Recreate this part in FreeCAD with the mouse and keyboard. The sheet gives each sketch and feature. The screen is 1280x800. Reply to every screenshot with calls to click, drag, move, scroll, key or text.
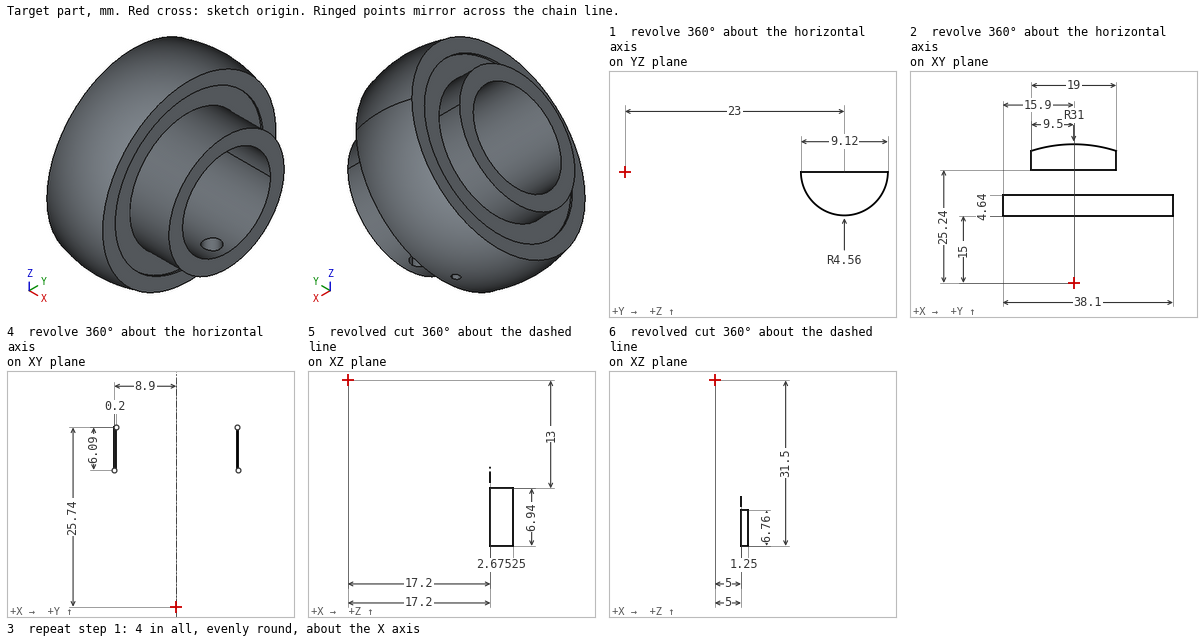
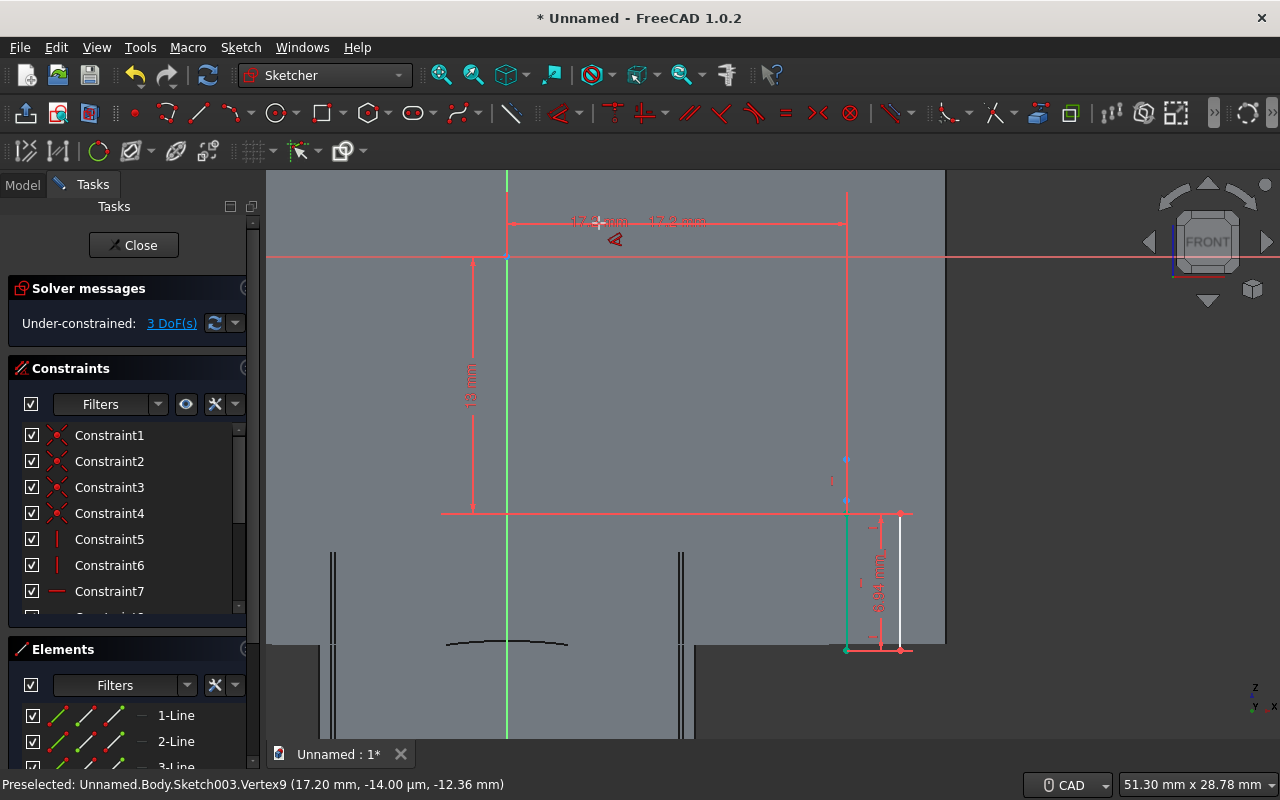
click(863, 651)
click(873, 685)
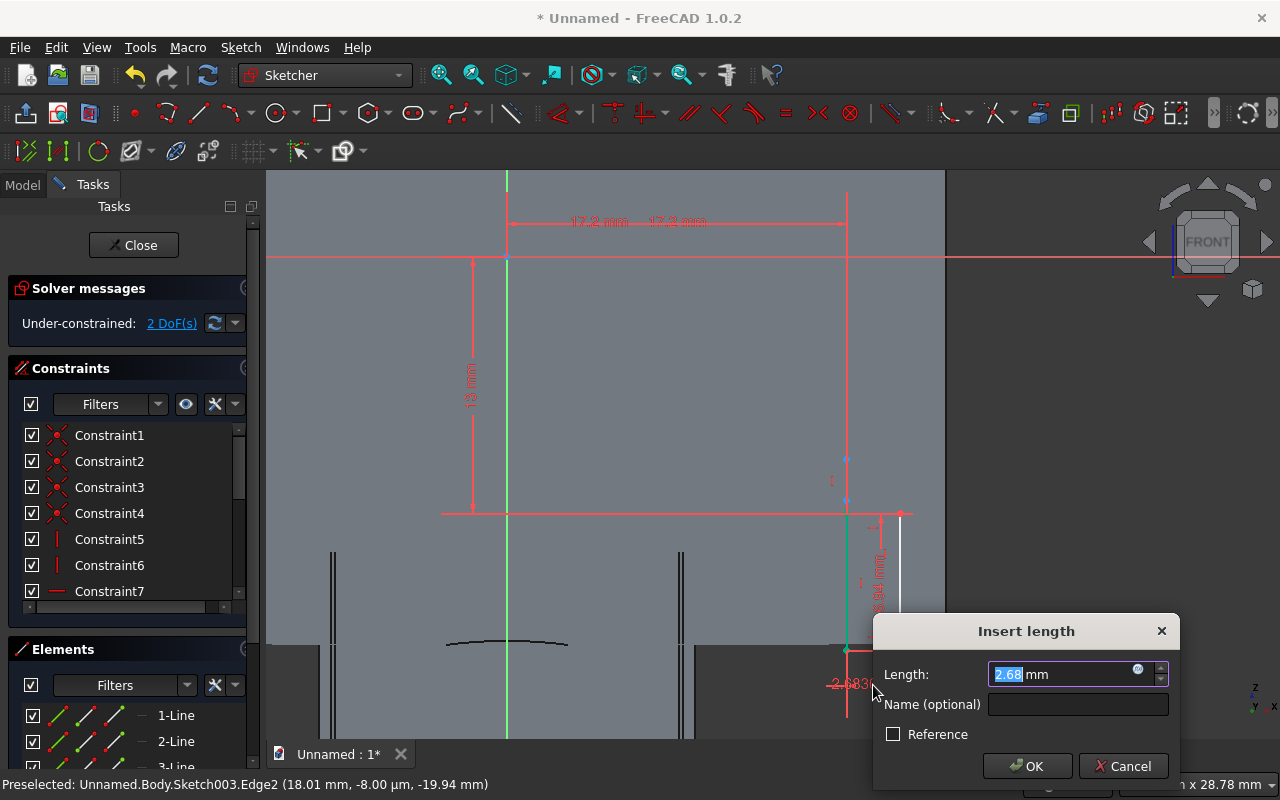
text(2.67525)
key(Return)
key(Escape)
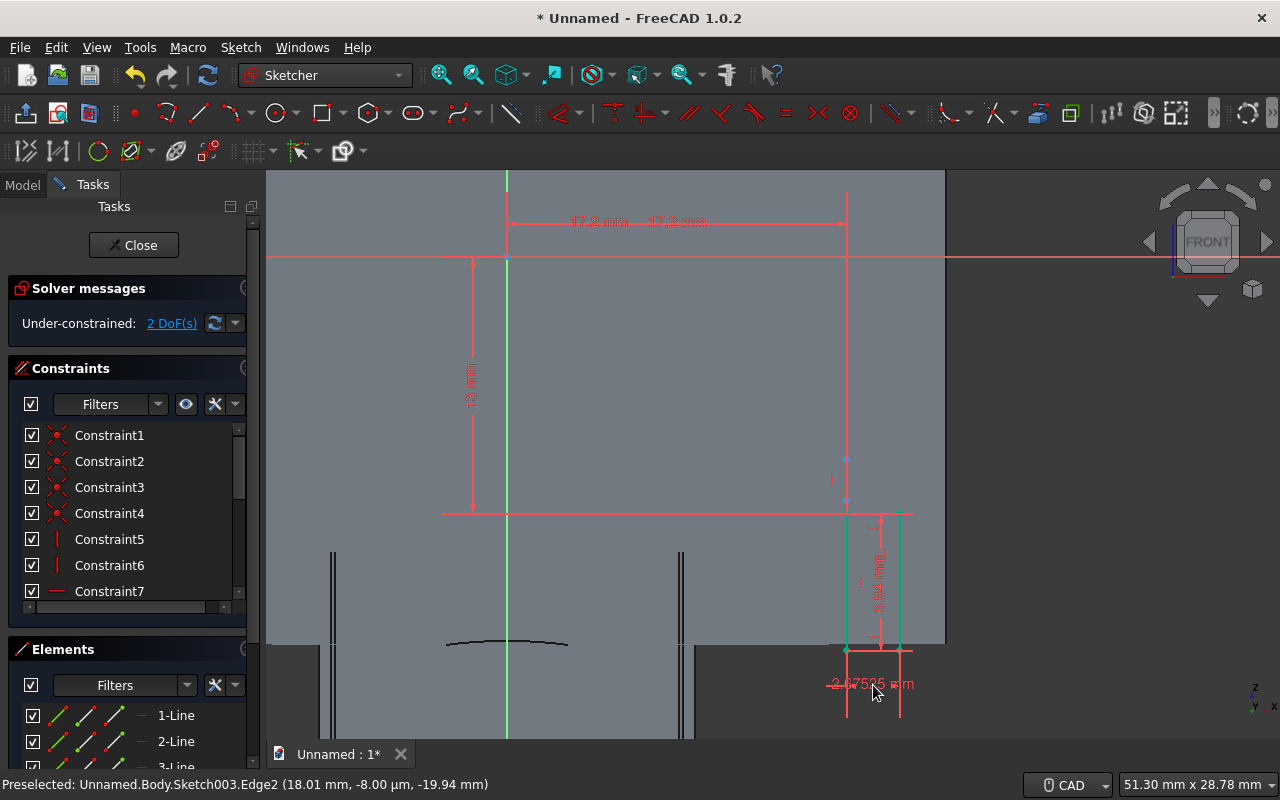
click(134, 245)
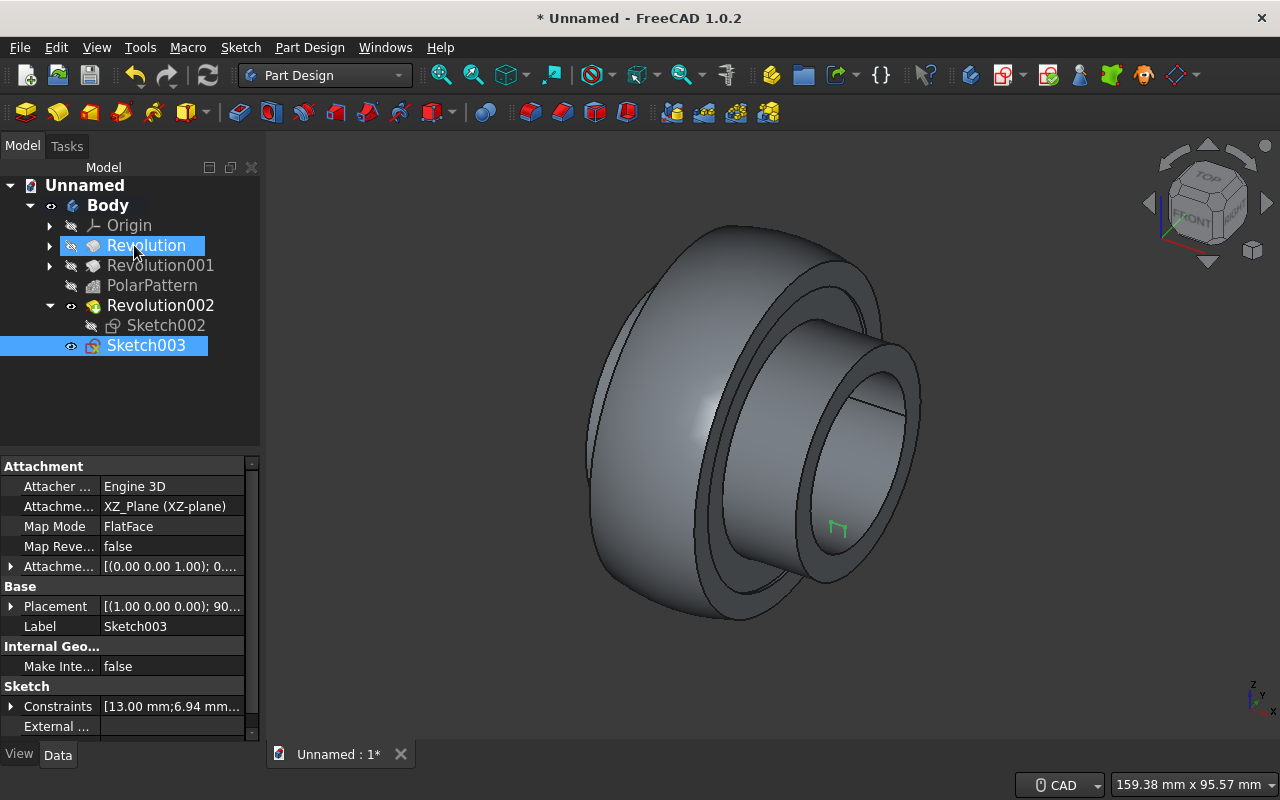
click(304, 112)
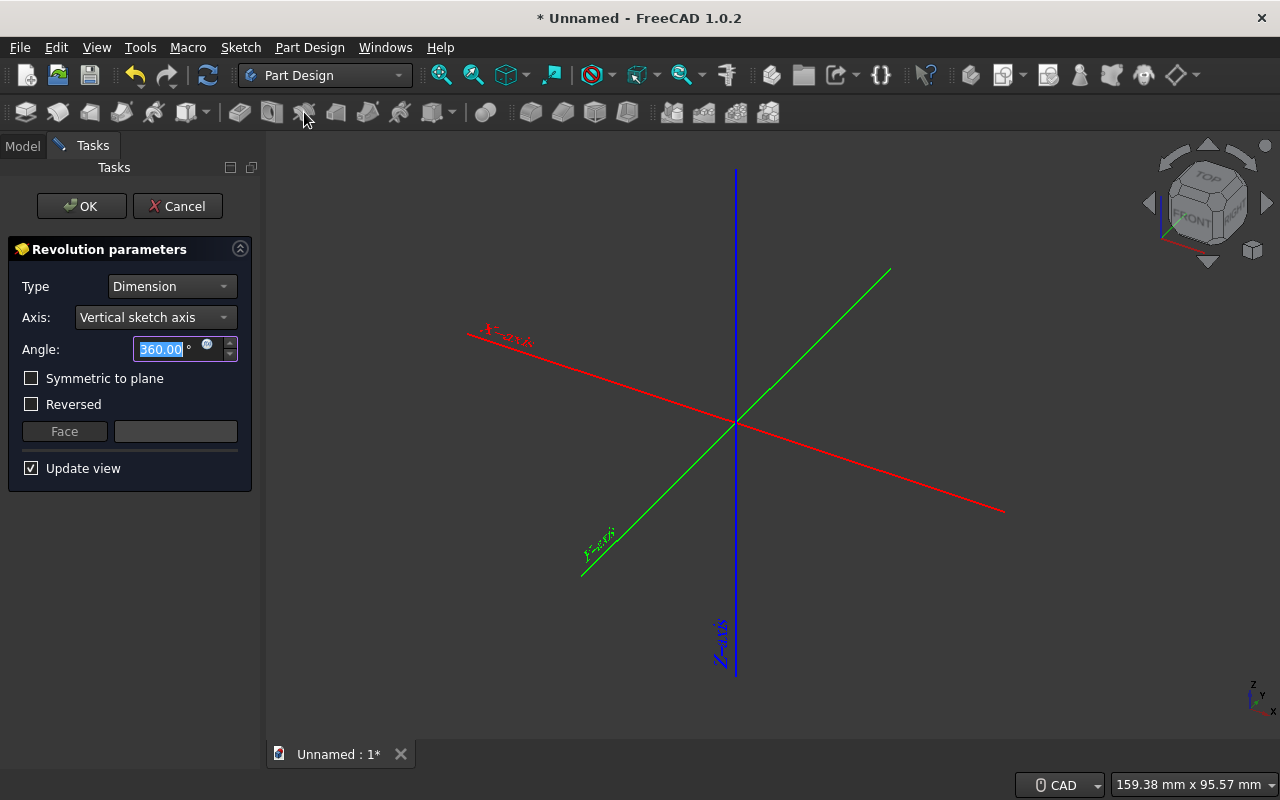
click(156, 318)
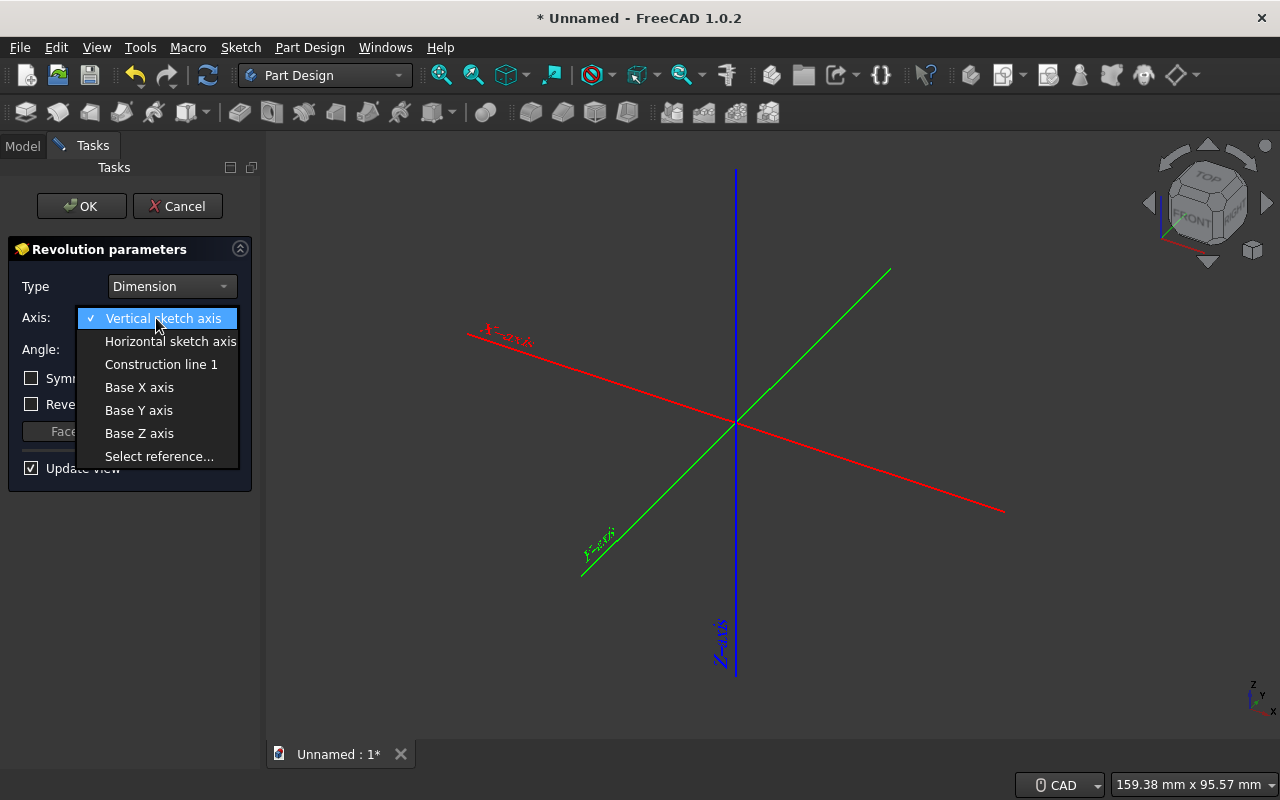
click(156, 364)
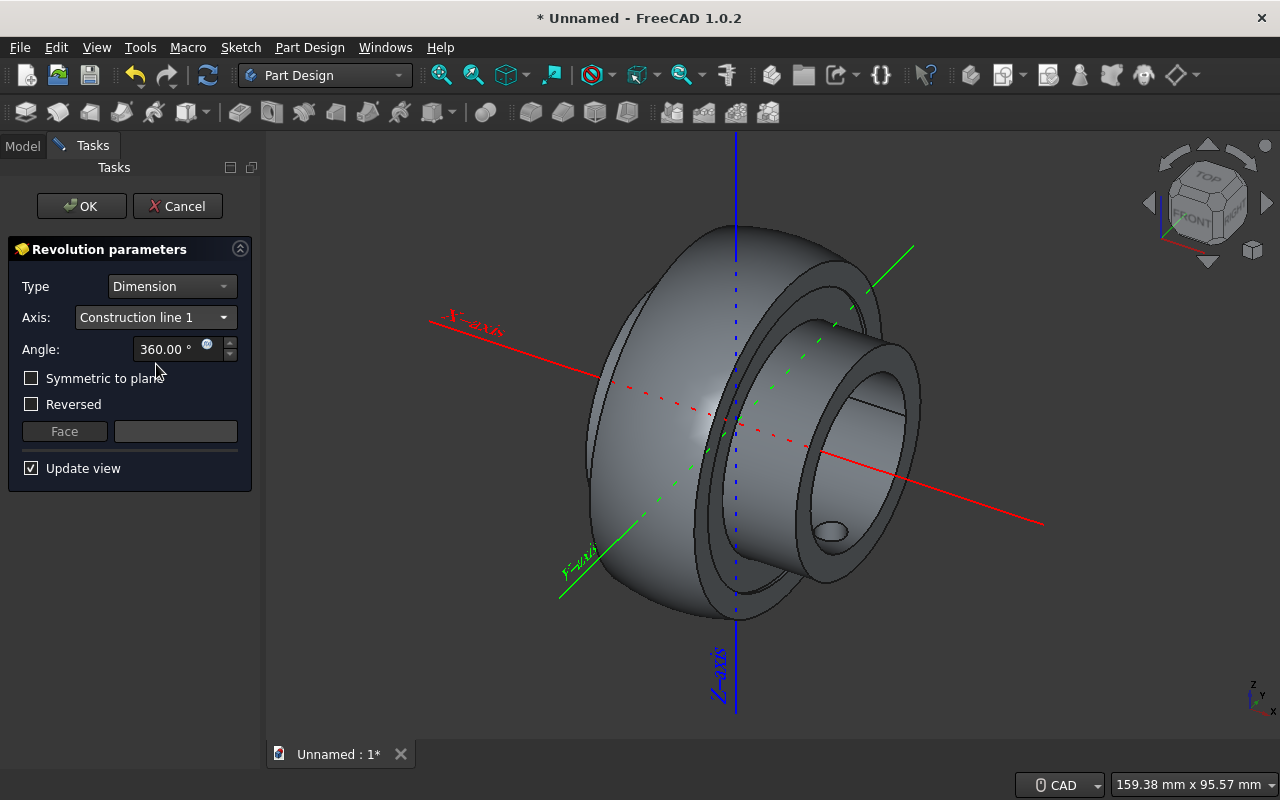
click(82, 206)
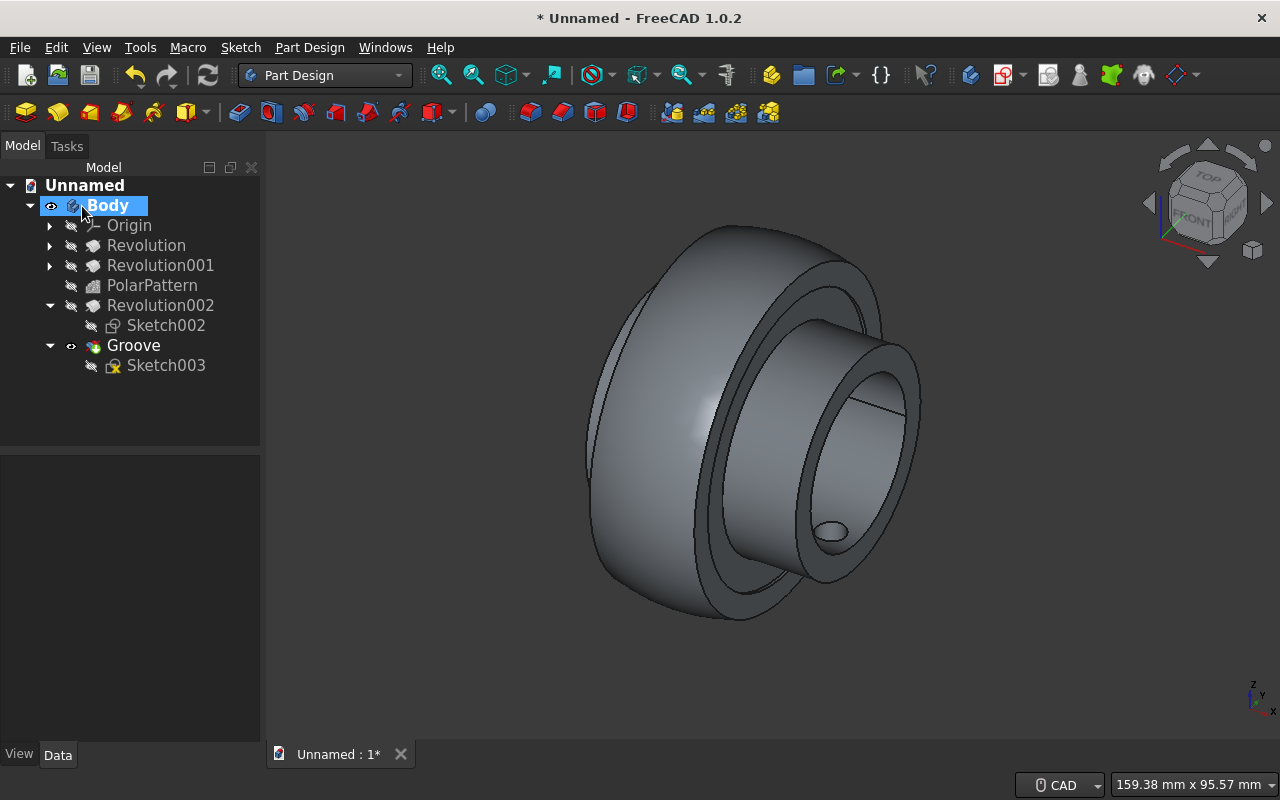
click(1004, 76)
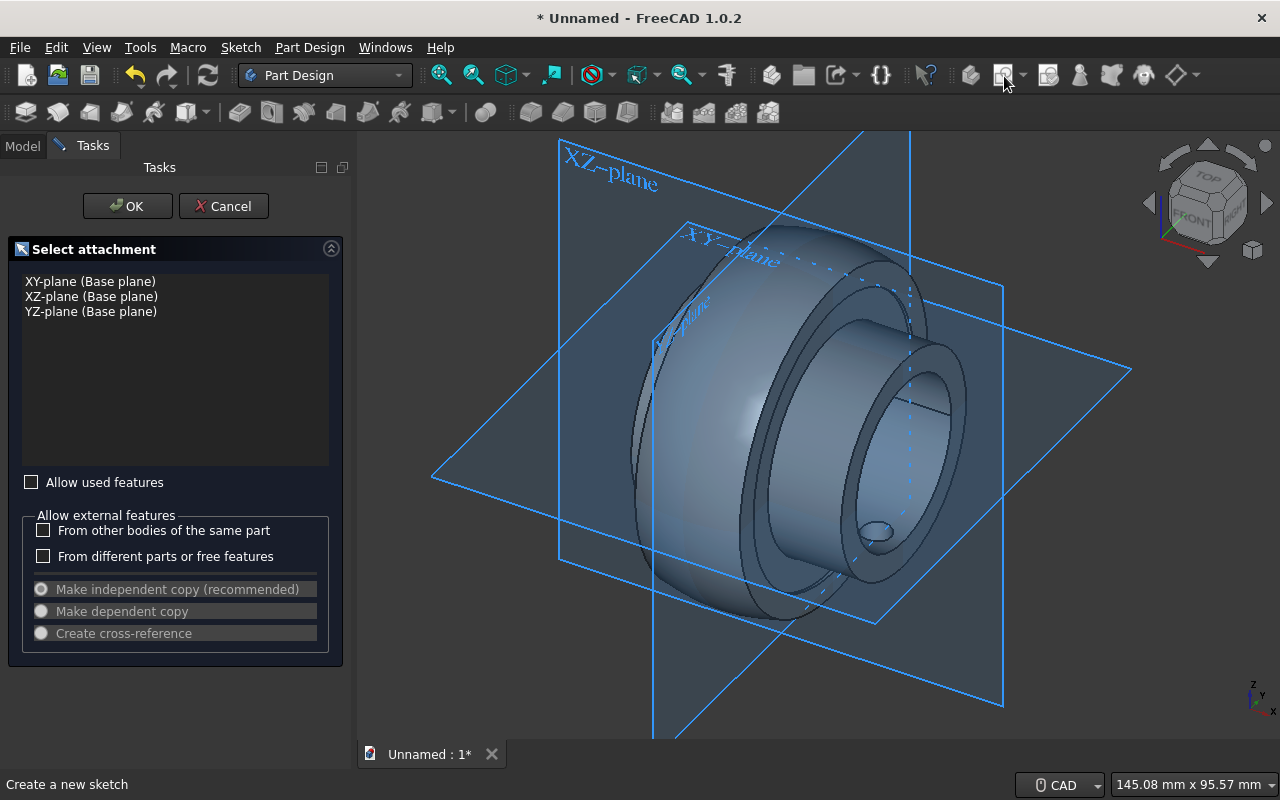
click(82, 296)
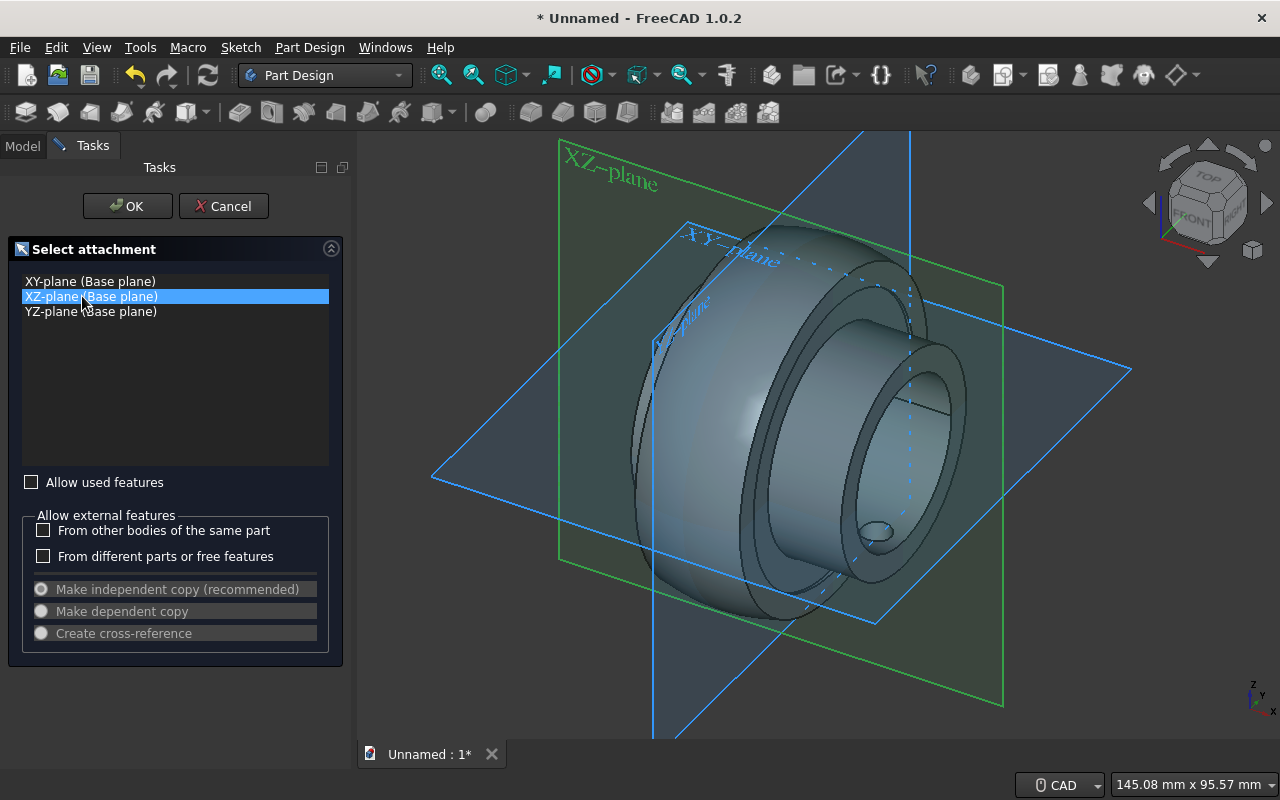
click(128, 206)